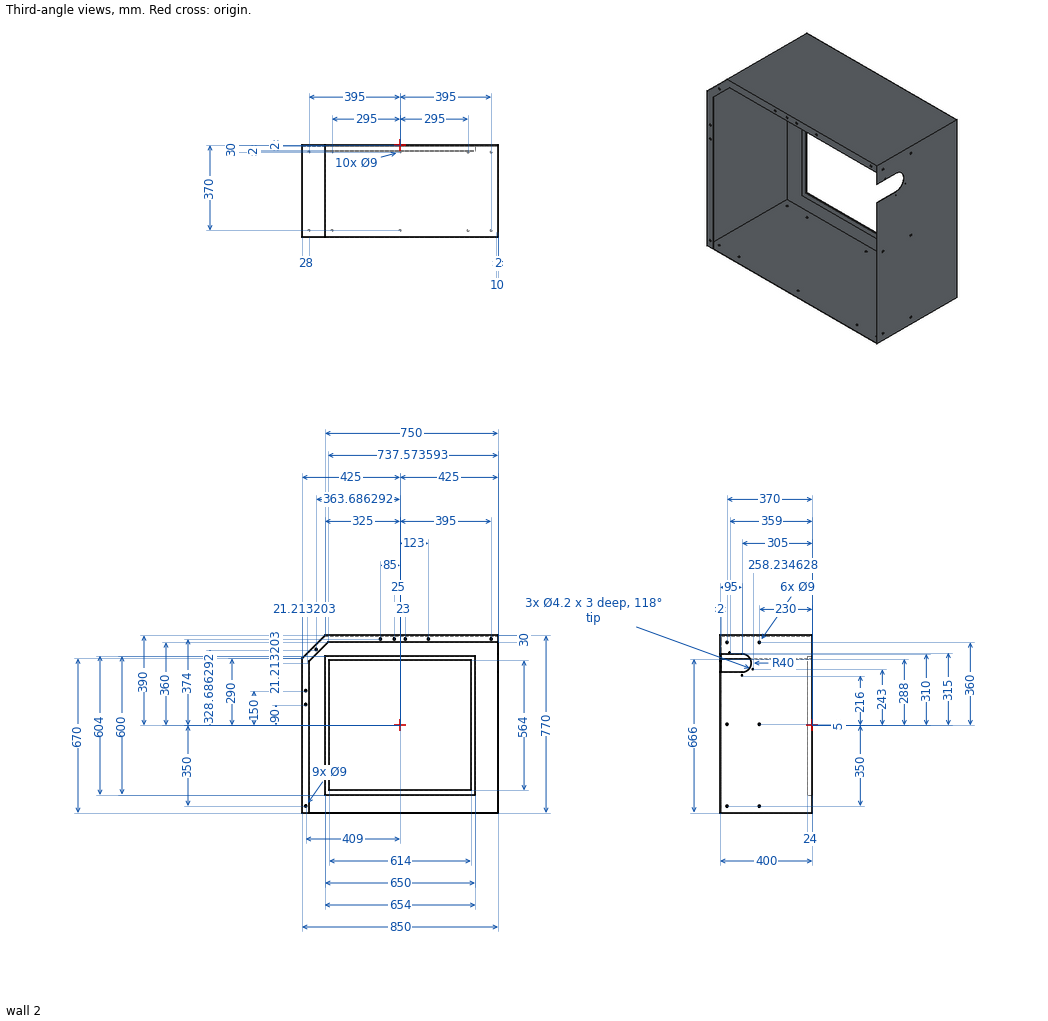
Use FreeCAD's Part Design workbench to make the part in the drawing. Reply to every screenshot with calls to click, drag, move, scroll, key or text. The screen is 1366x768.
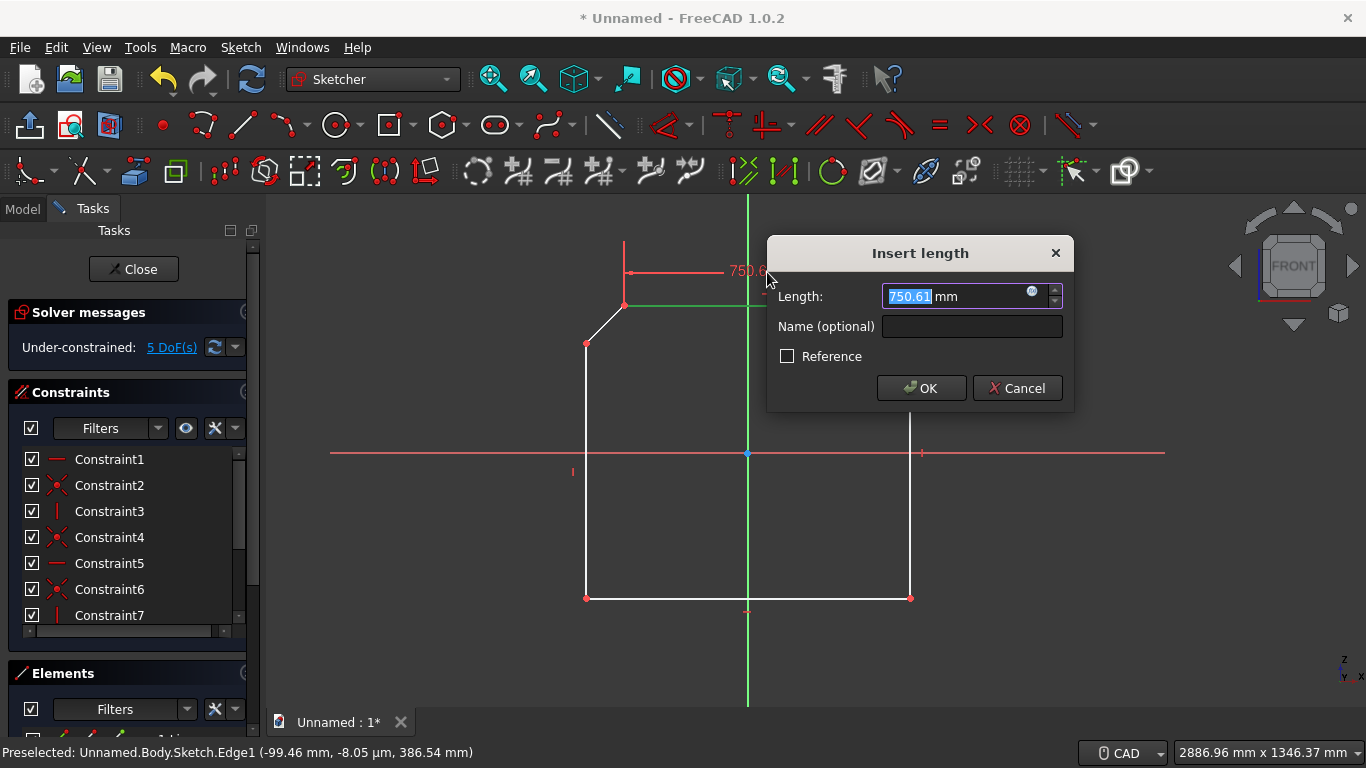
text(750)
key(Return)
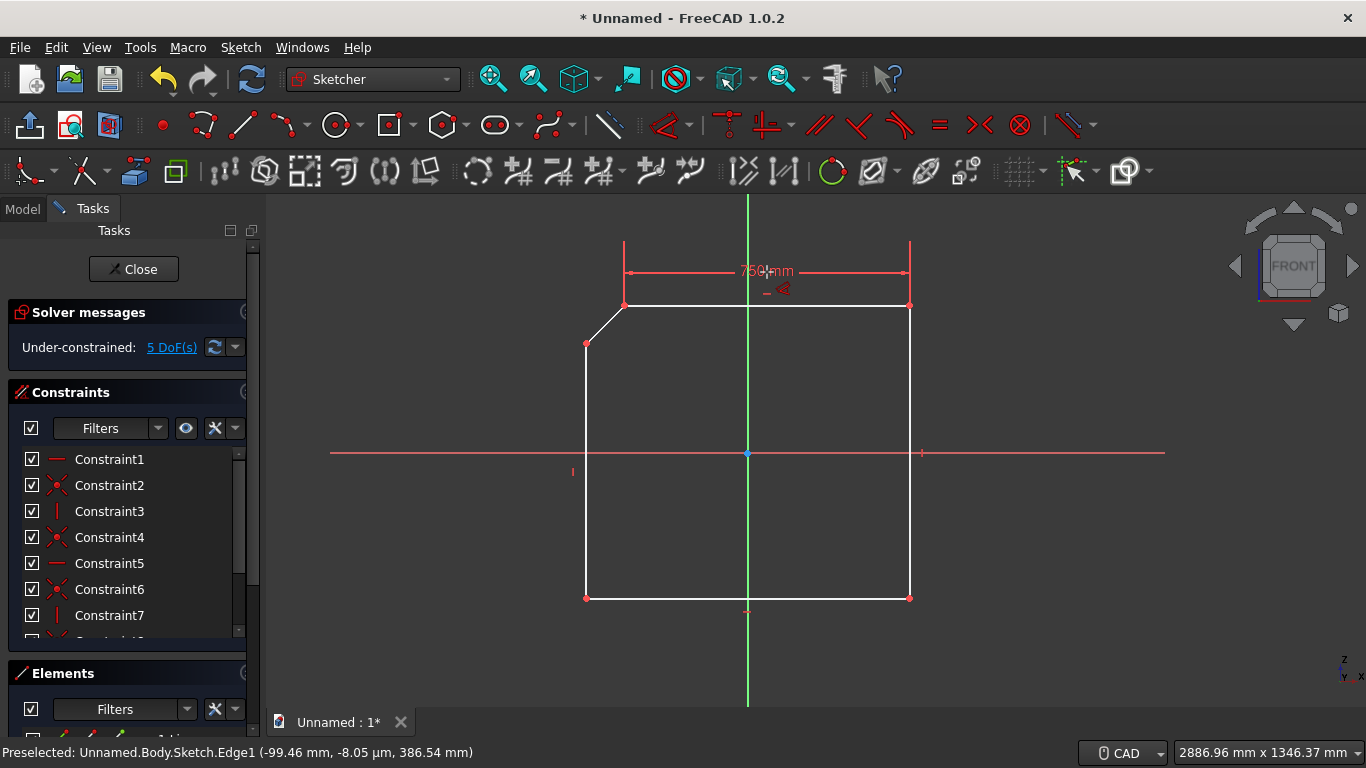
click(910, 394)
click(944, 385)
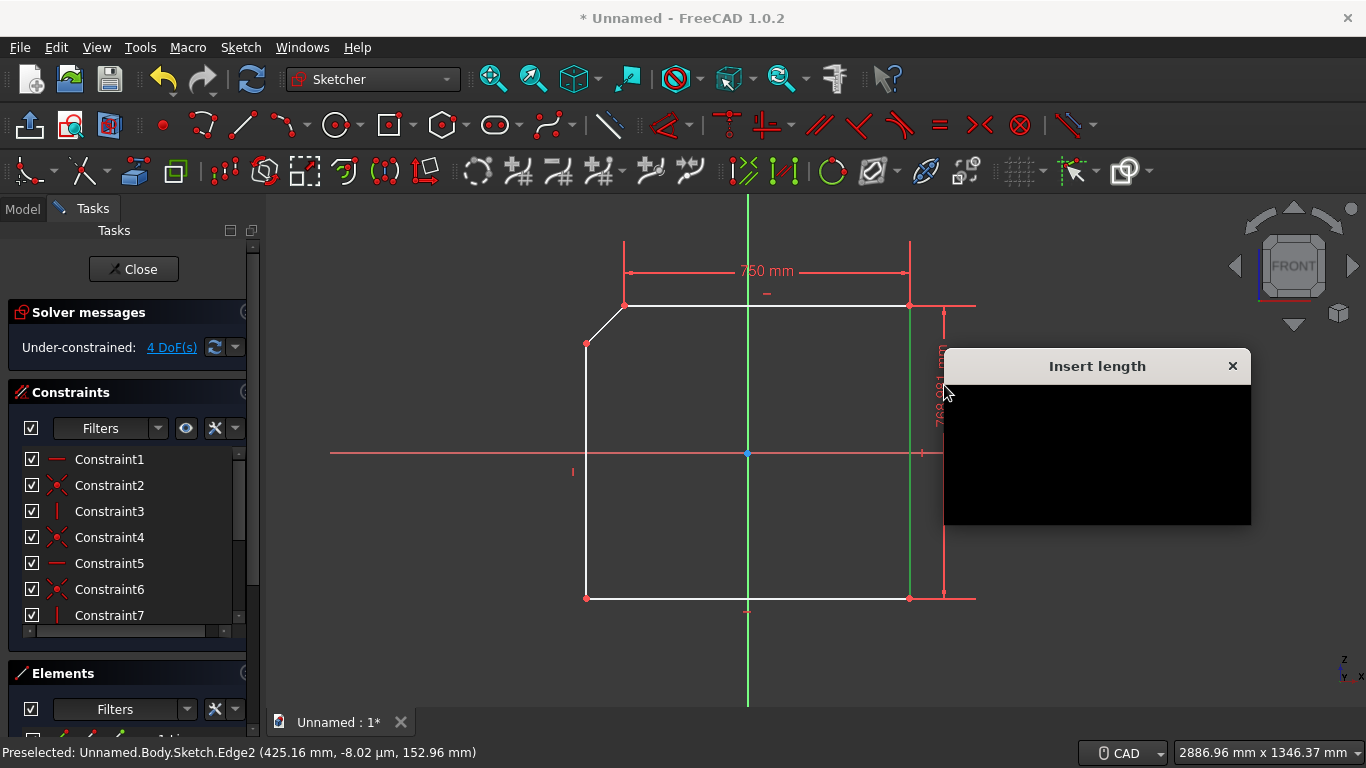
text(770)
key(Return)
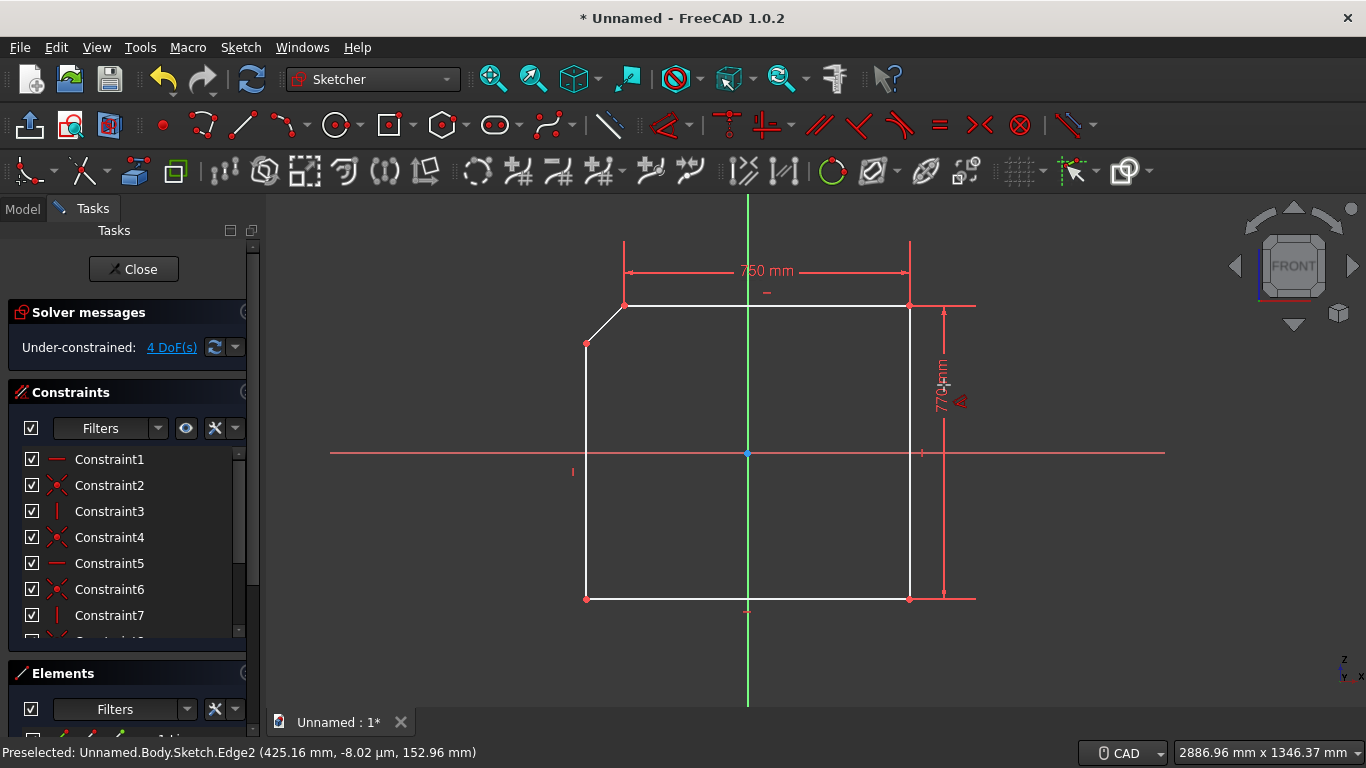
click(813, 599)
click(673, 633)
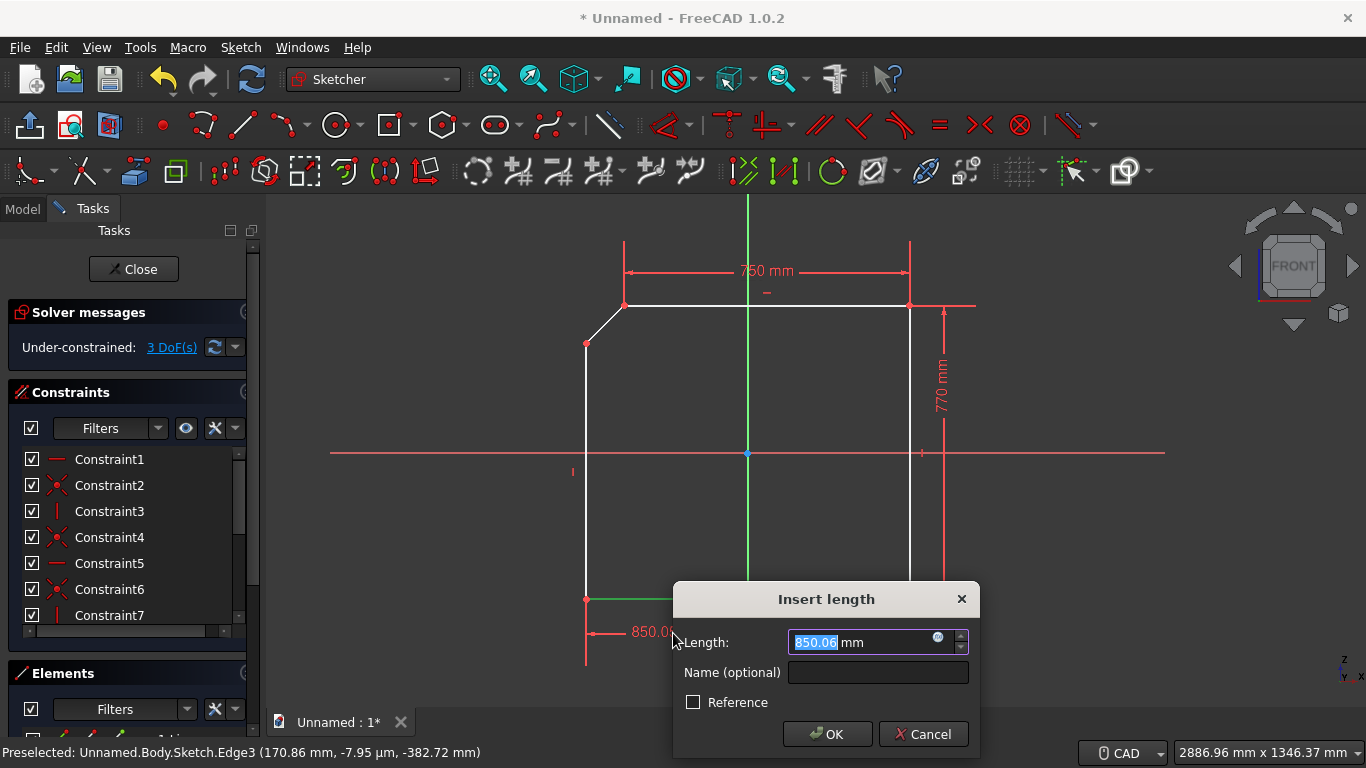
text(850)
key(Return)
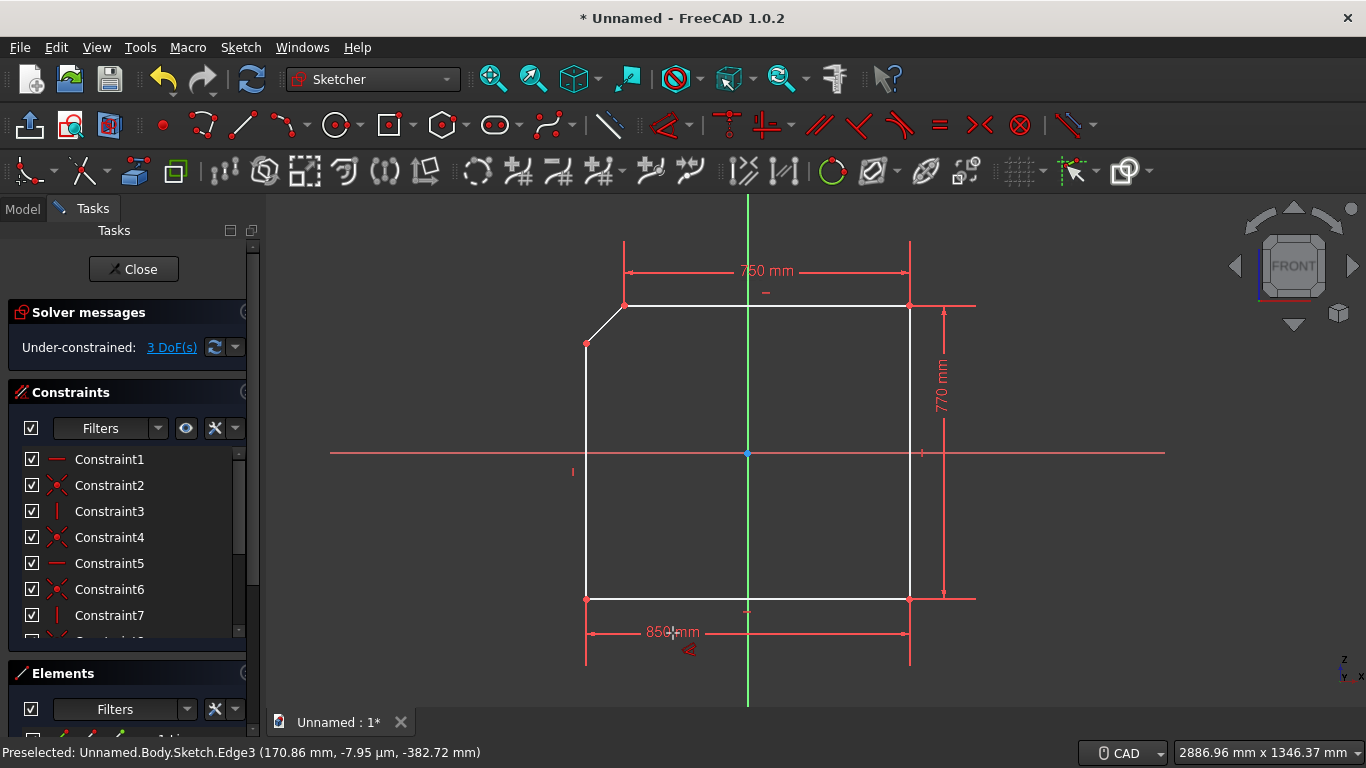
click(586, 523)
click(552, 472)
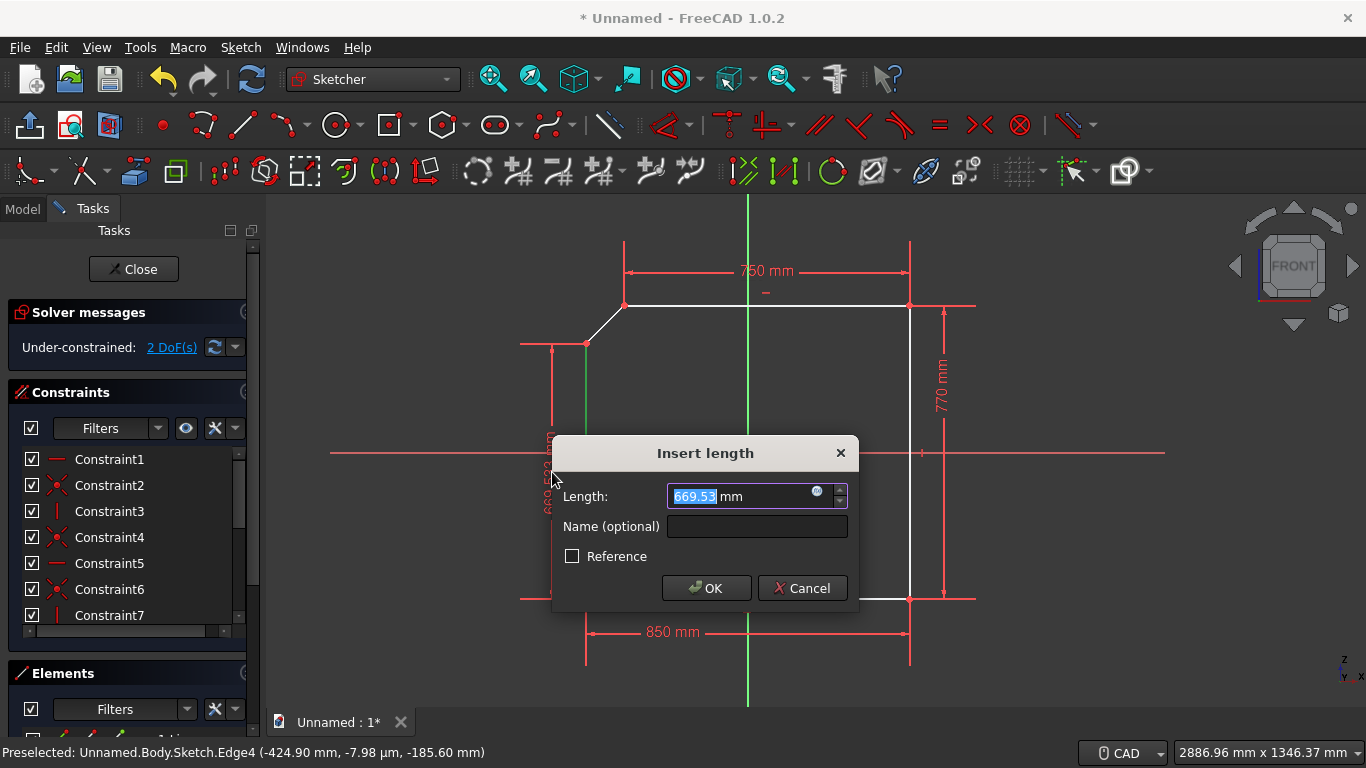
text(670)
key(Return)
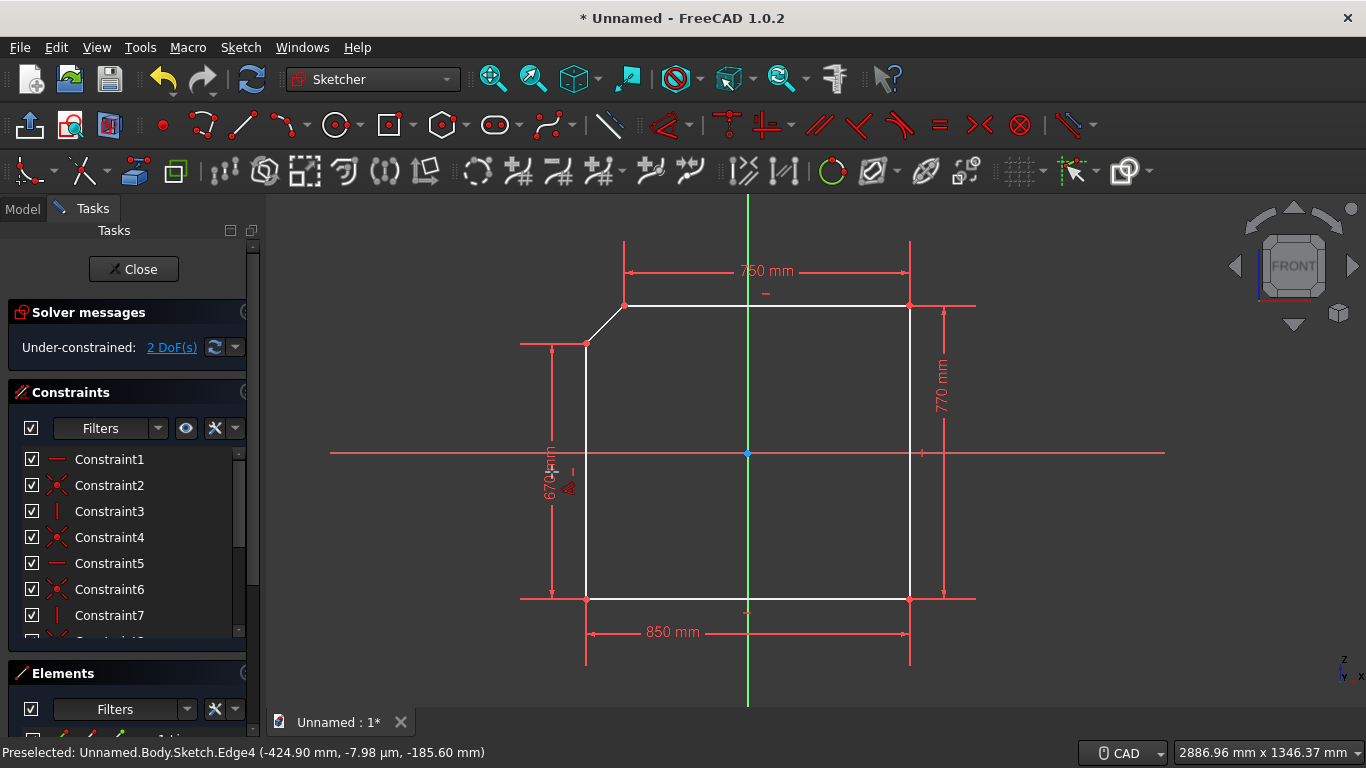
click(624, 306)
click(686, 272)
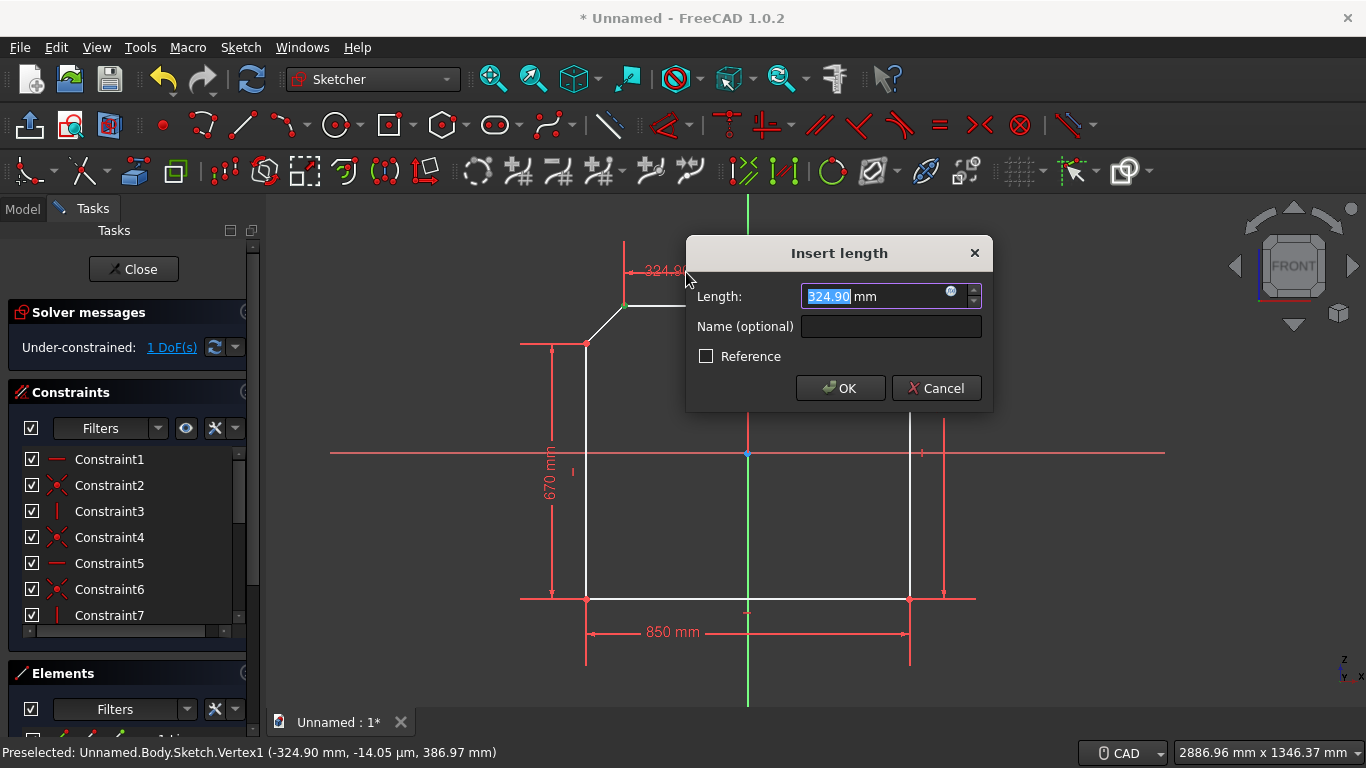
text(325)
key(Return)